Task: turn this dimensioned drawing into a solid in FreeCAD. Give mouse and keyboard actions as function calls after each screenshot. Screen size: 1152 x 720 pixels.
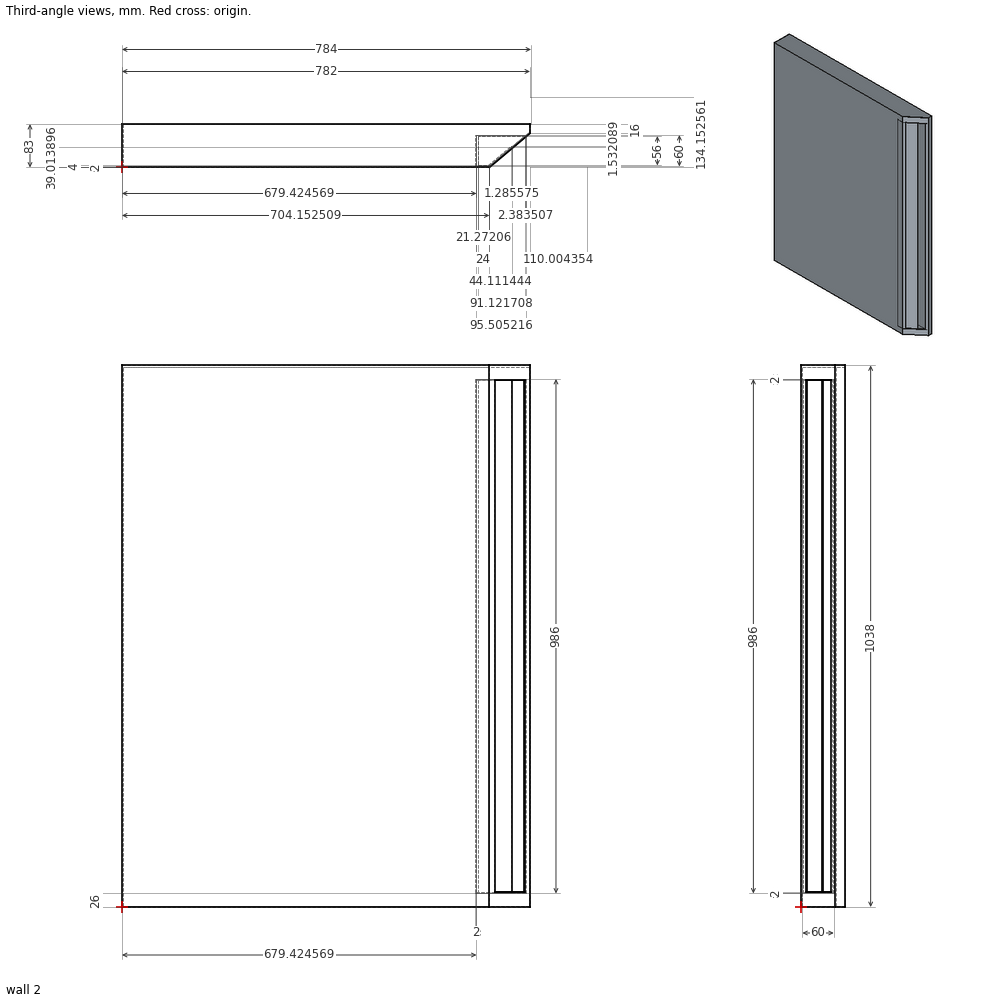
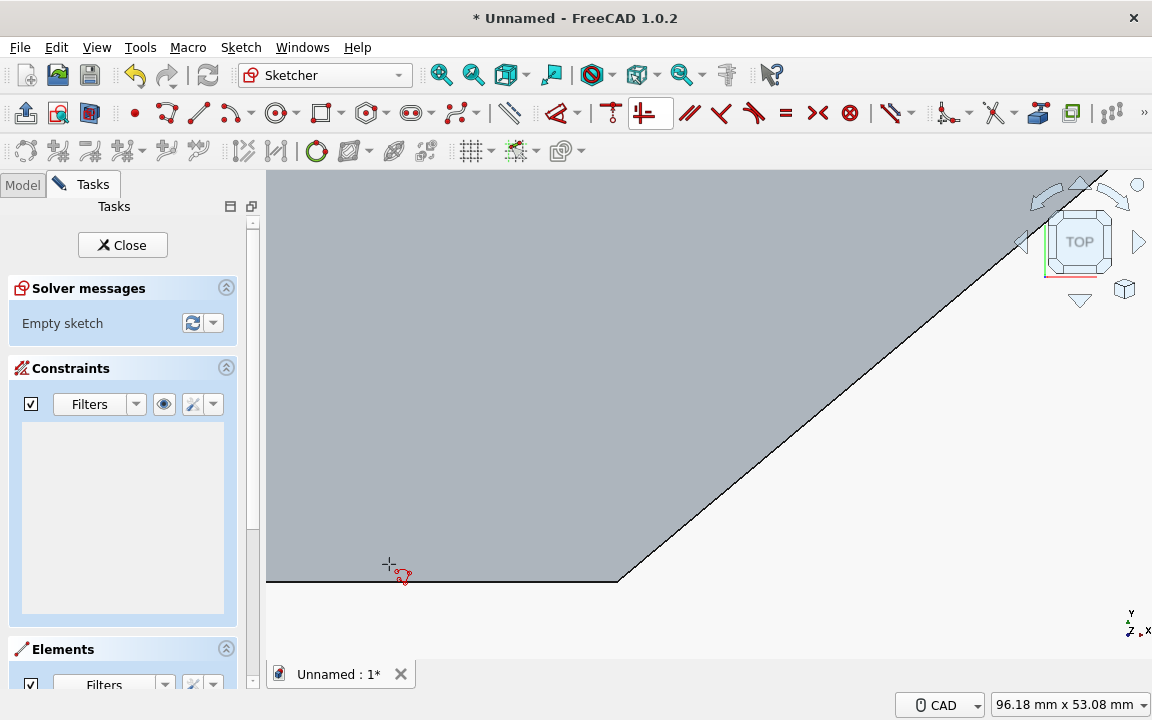
click(389, 564)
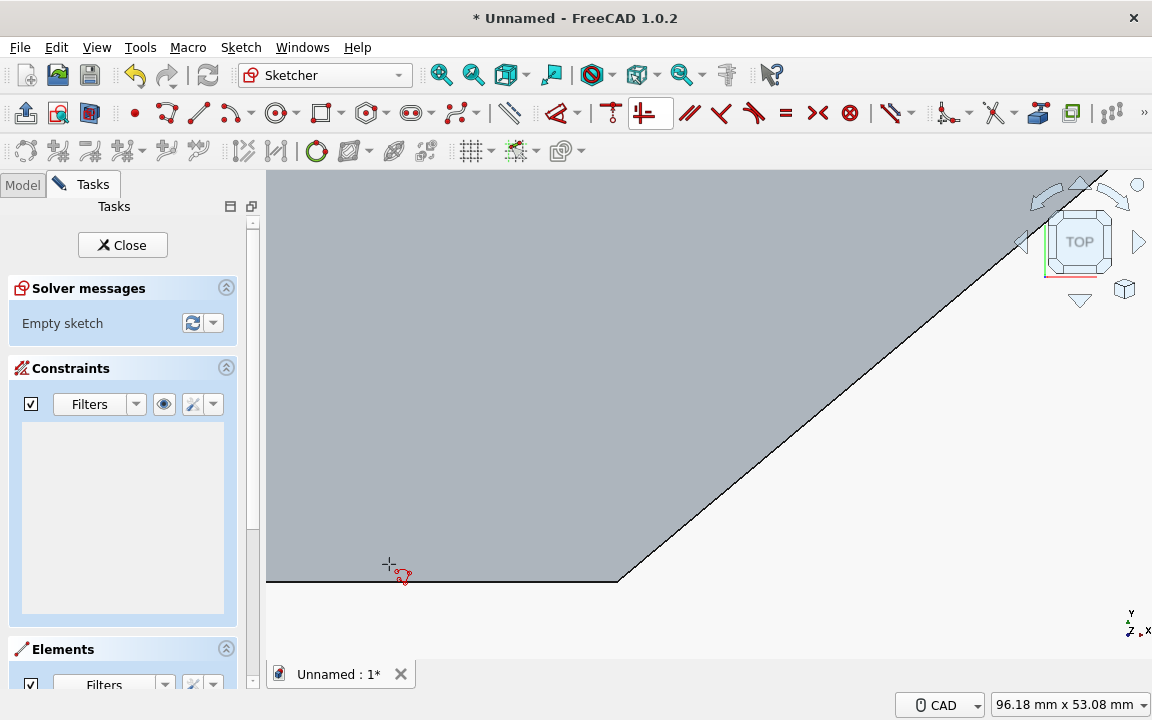
scroll(411, 569, down, 3)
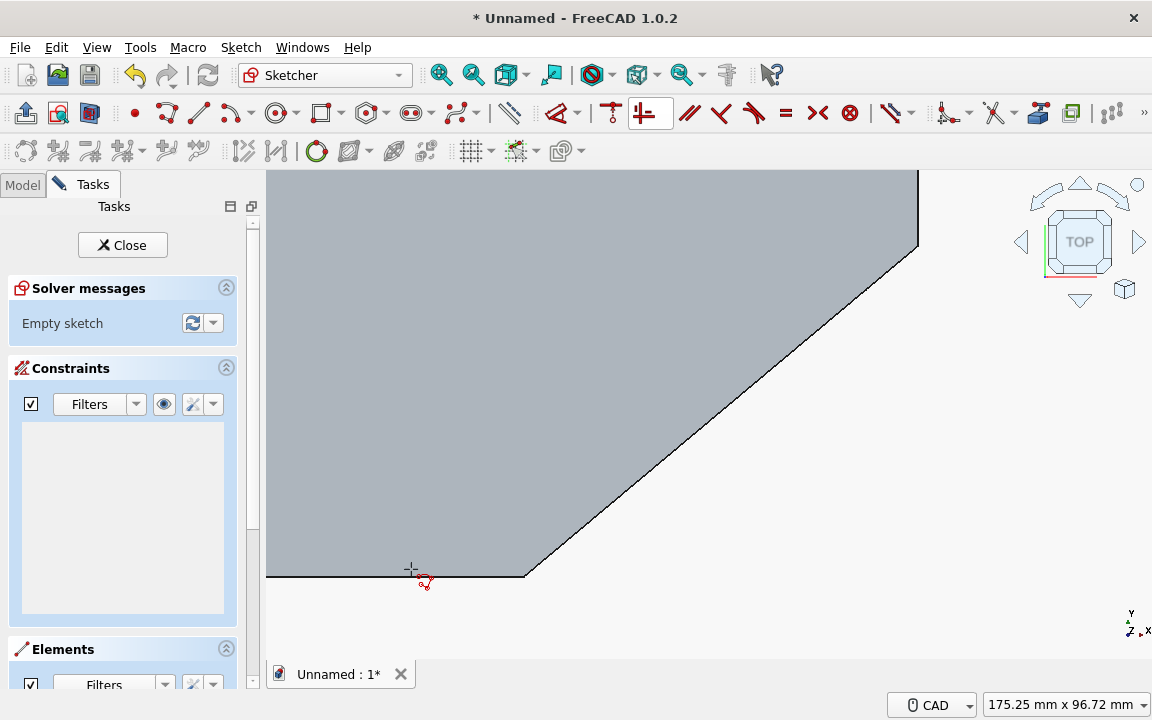
click(399, 263)
click(882, 263)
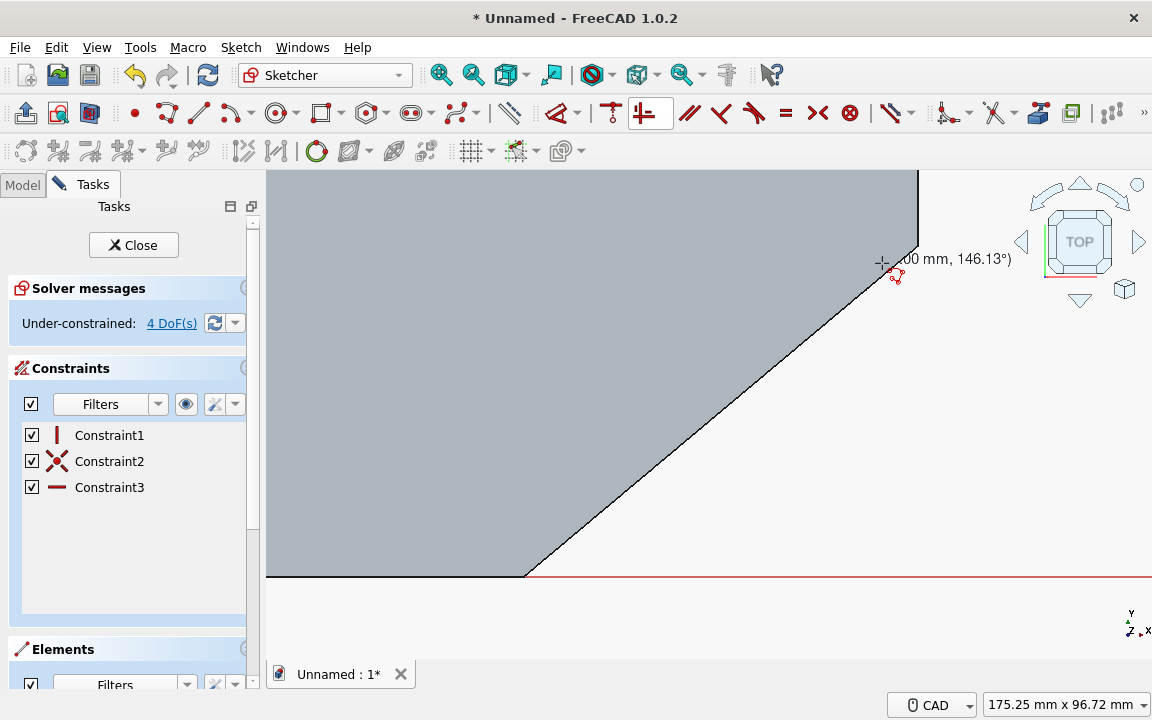
scroll(520, 567, up, 3)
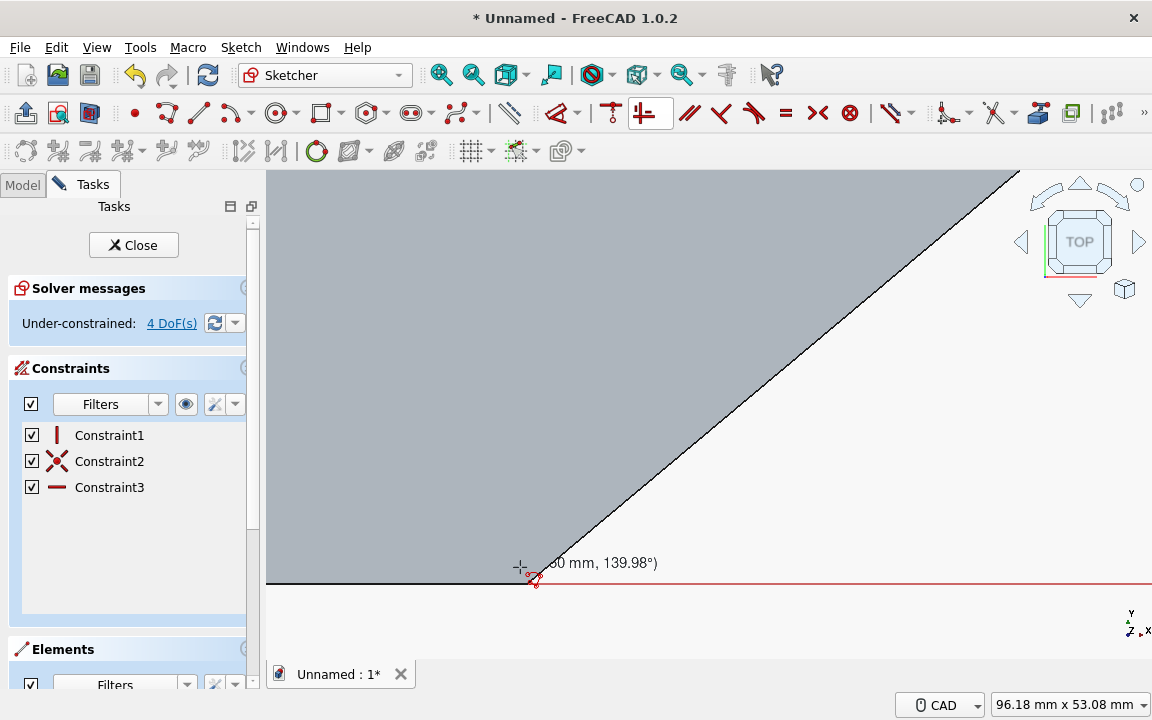
click(520, 565)
click(299, 567)
key(Escape)
key(Escape)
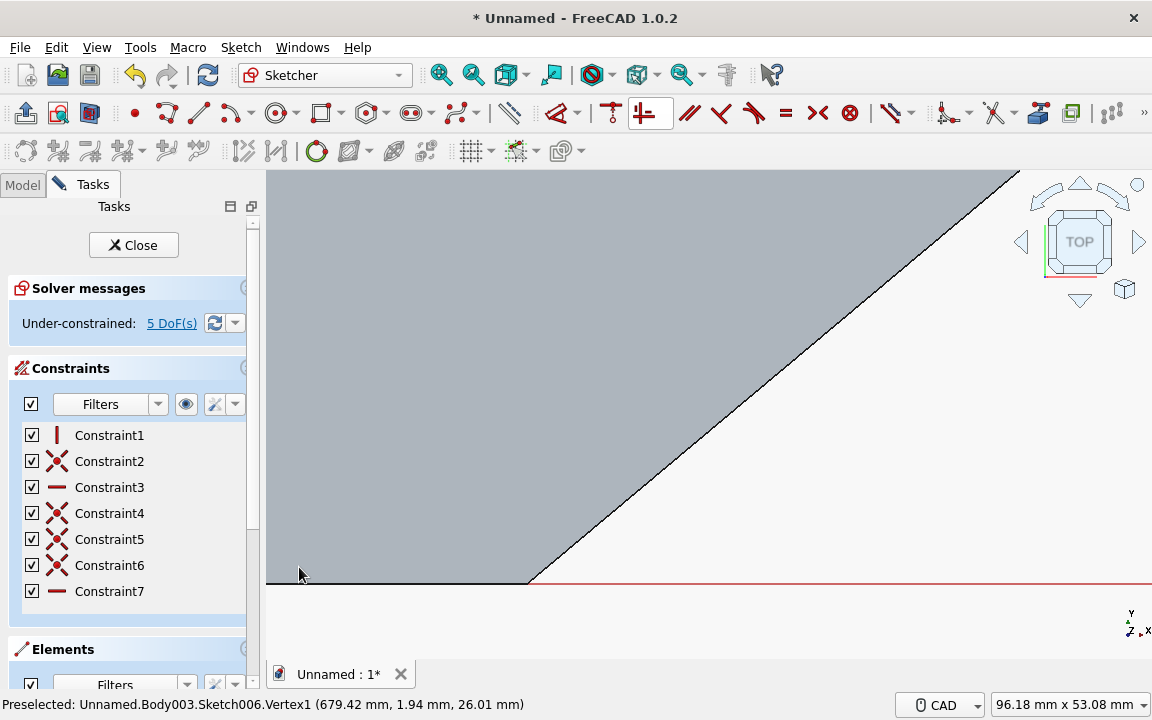
key(d)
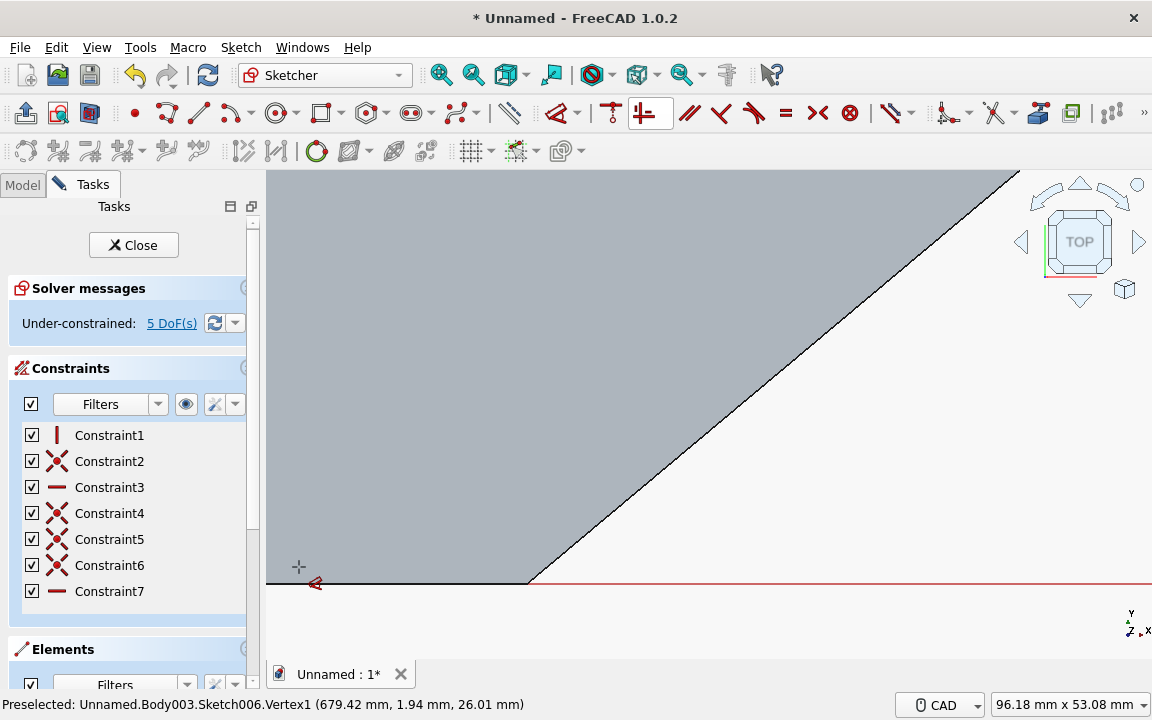
click(299, 400)
click(333, 382)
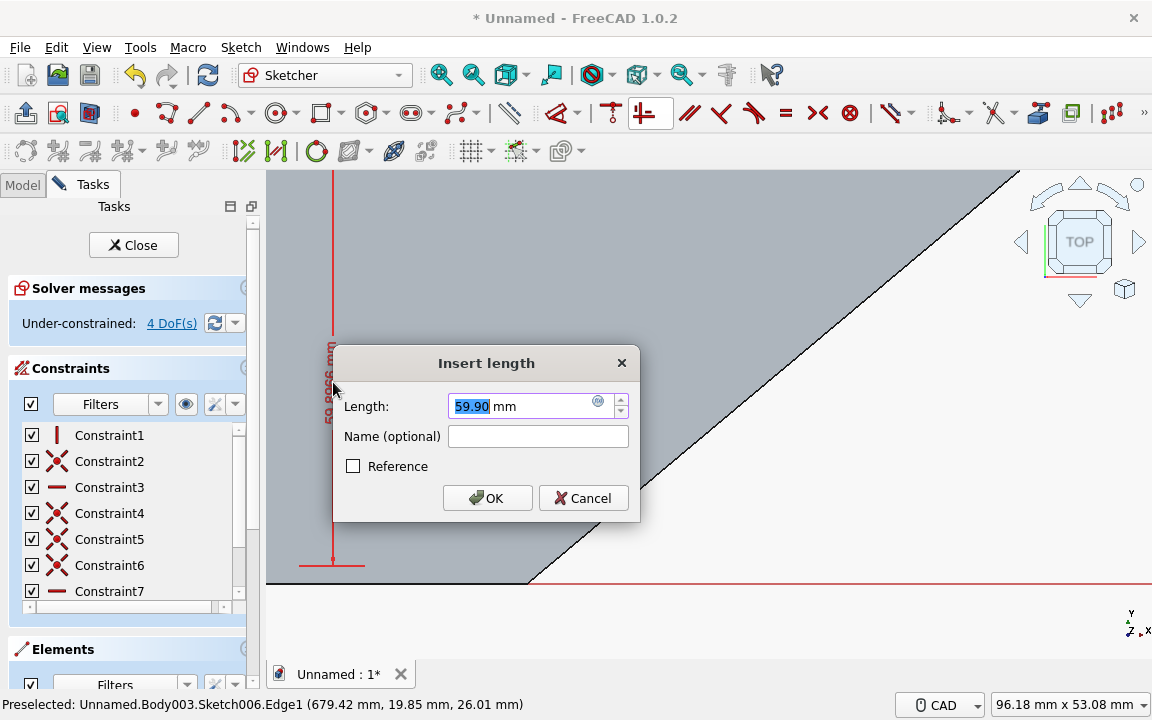
text(60)
key(Return)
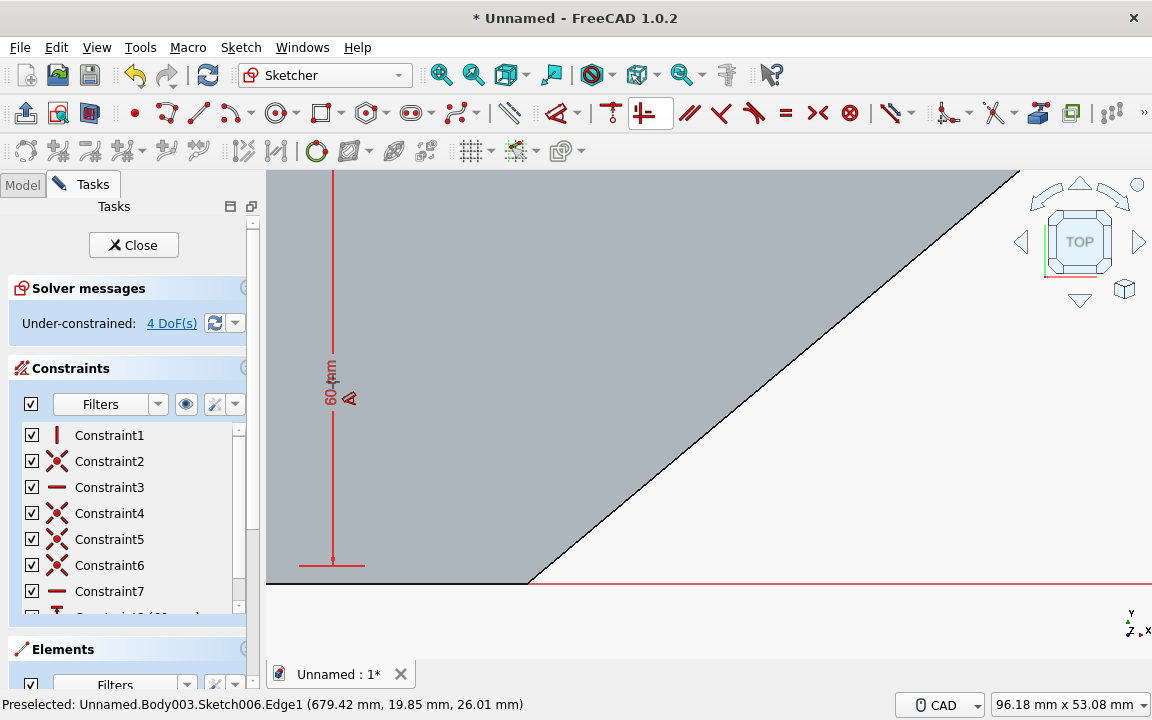
click(454, 566)
click(410, 600)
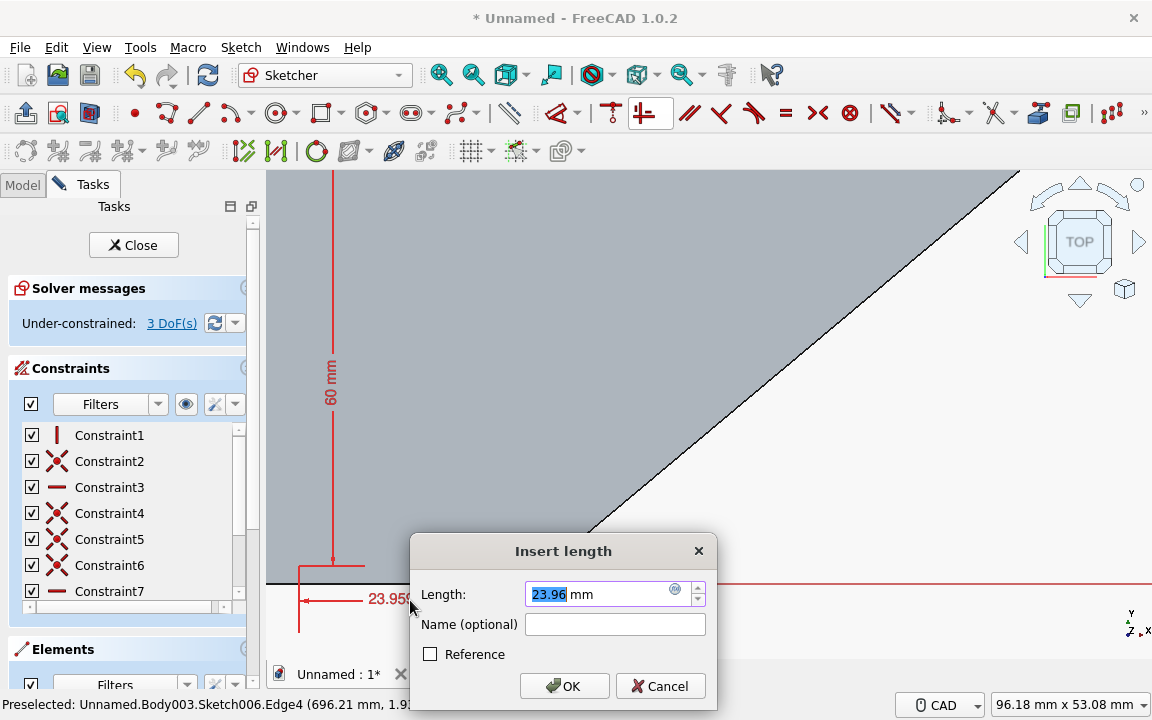
text(24)
key(Return)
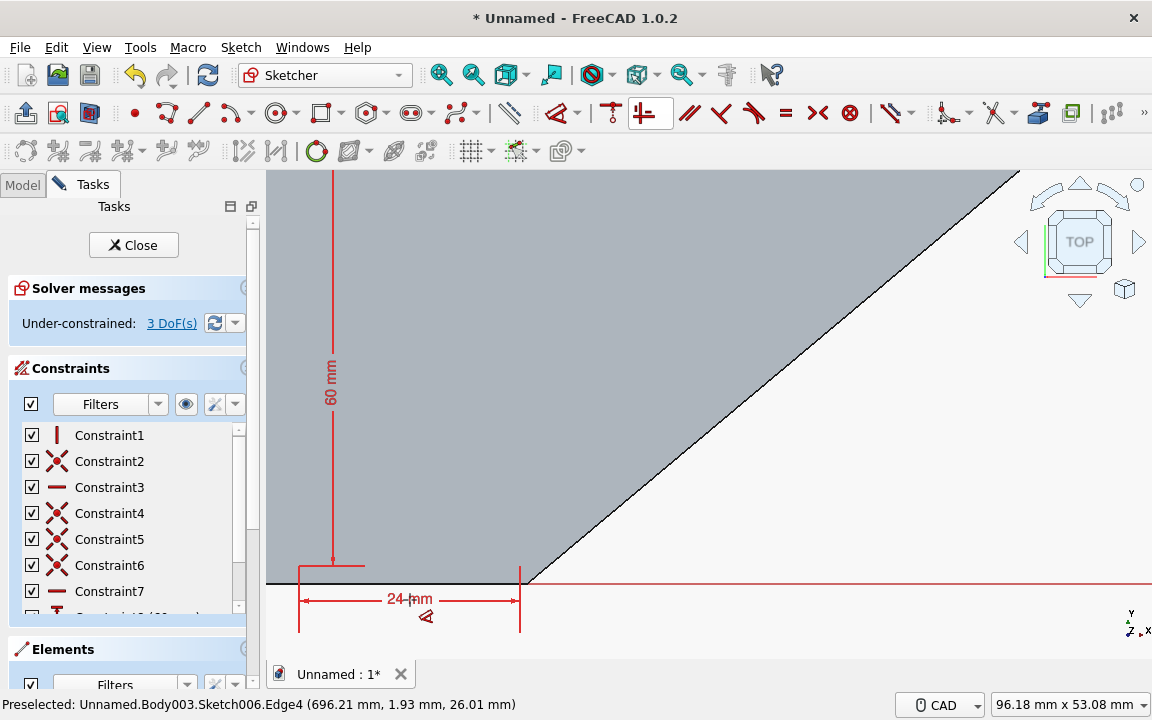
scroll(299, 566, up, 4)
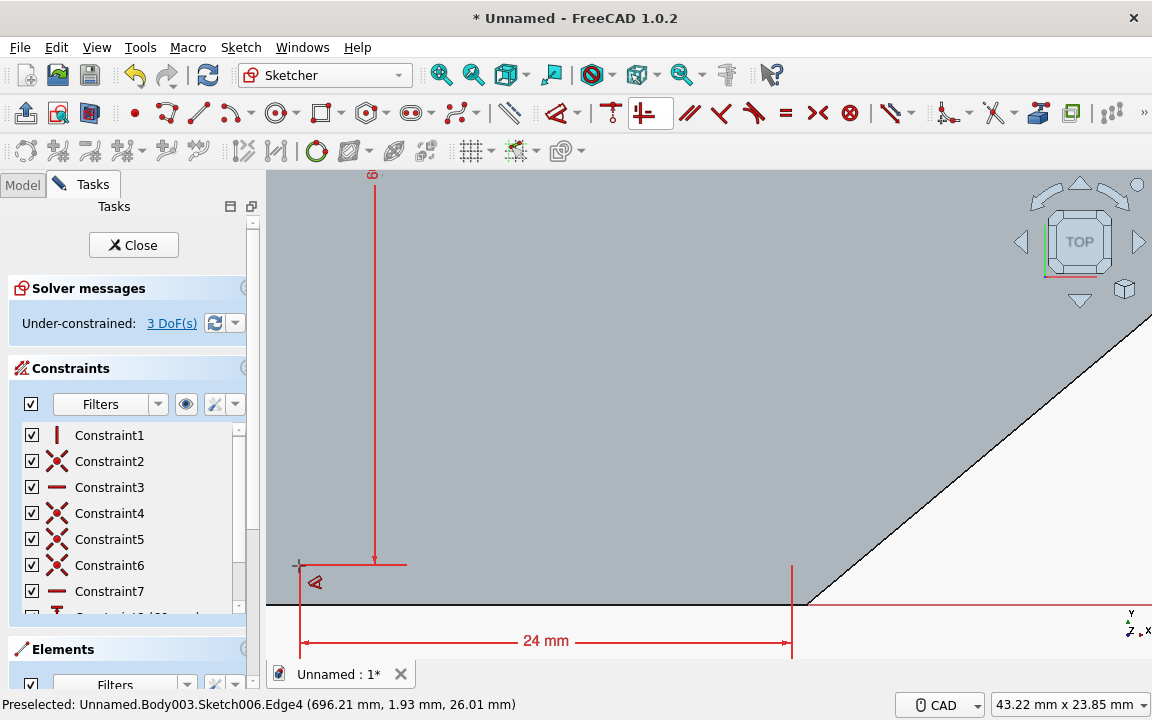
click(300, 565)
click(334, 585)